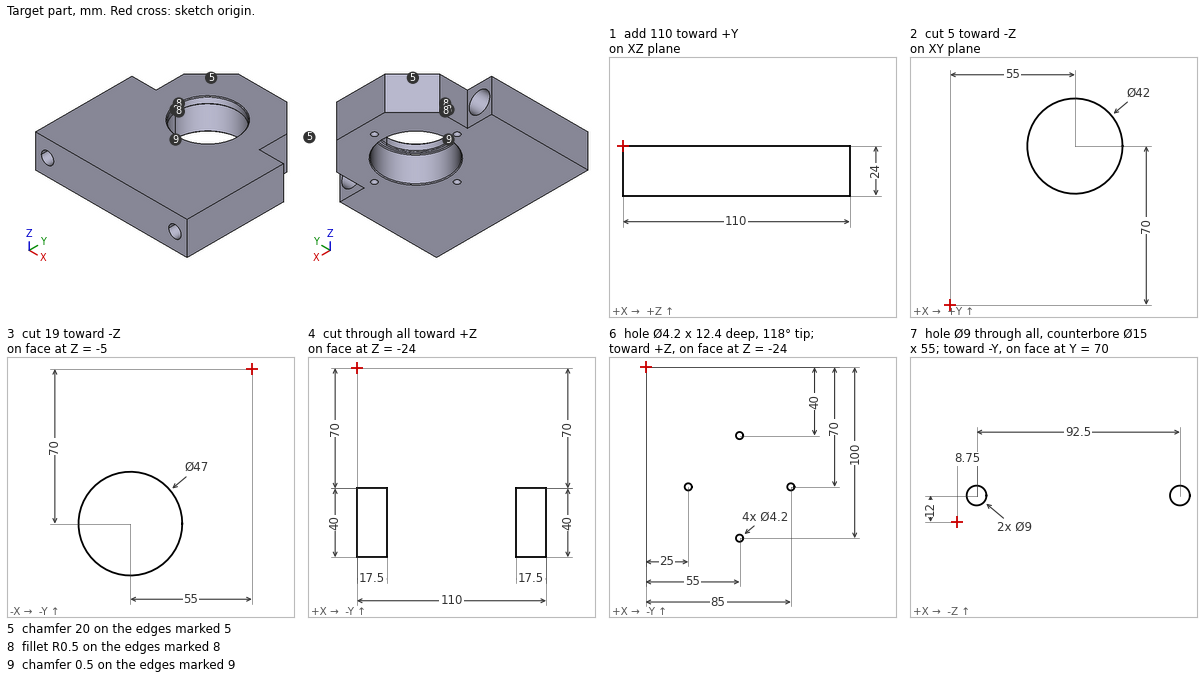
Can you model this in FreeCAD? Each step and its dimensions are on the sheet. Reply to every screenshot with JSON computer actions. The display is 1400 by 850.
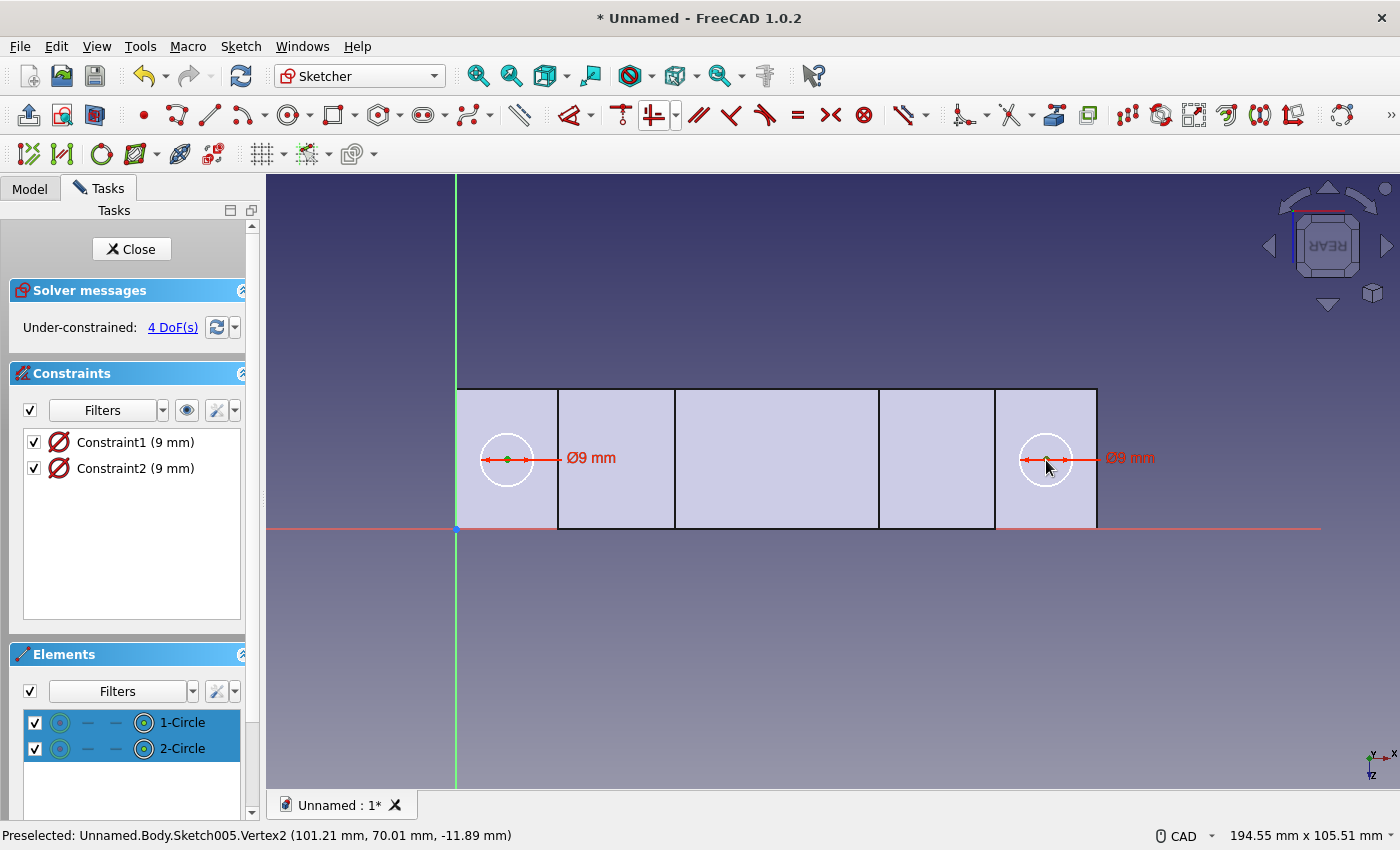
{"action": "left_click", "coordinate": [676, 116]}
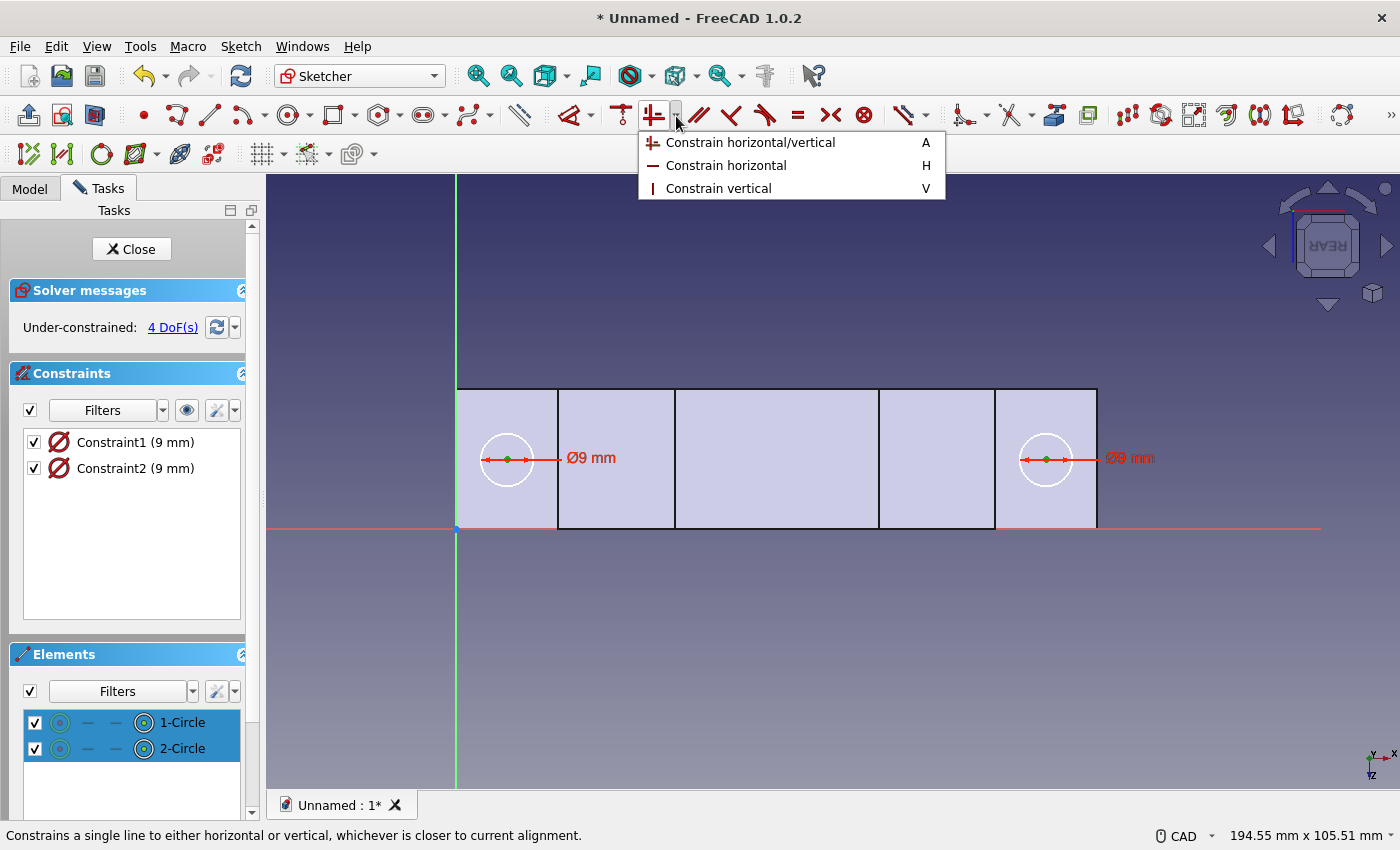
{"action": "left_click", "coordinate": [792, 166]}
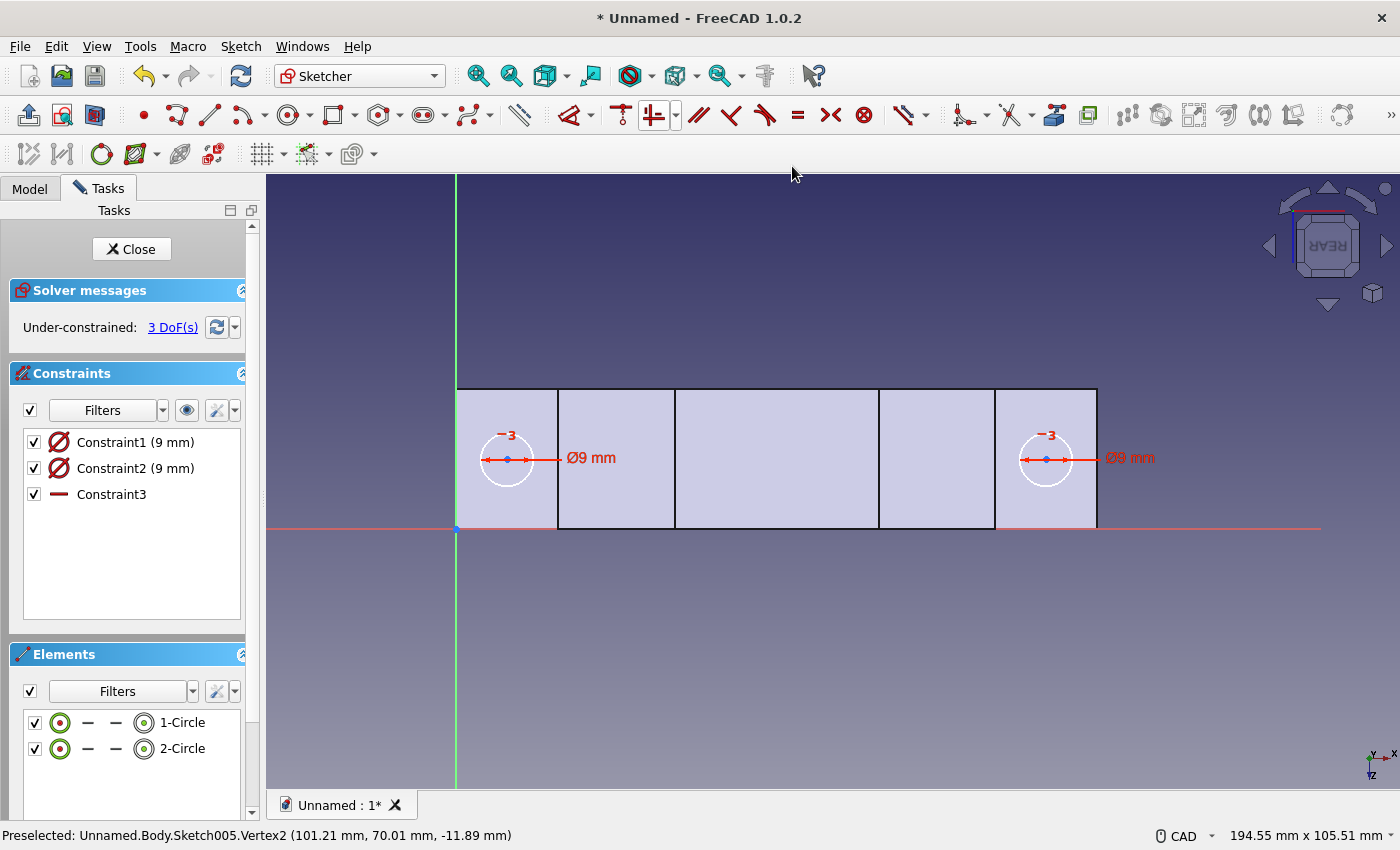
{"action": "left_click", "coordinate": [568, 116]}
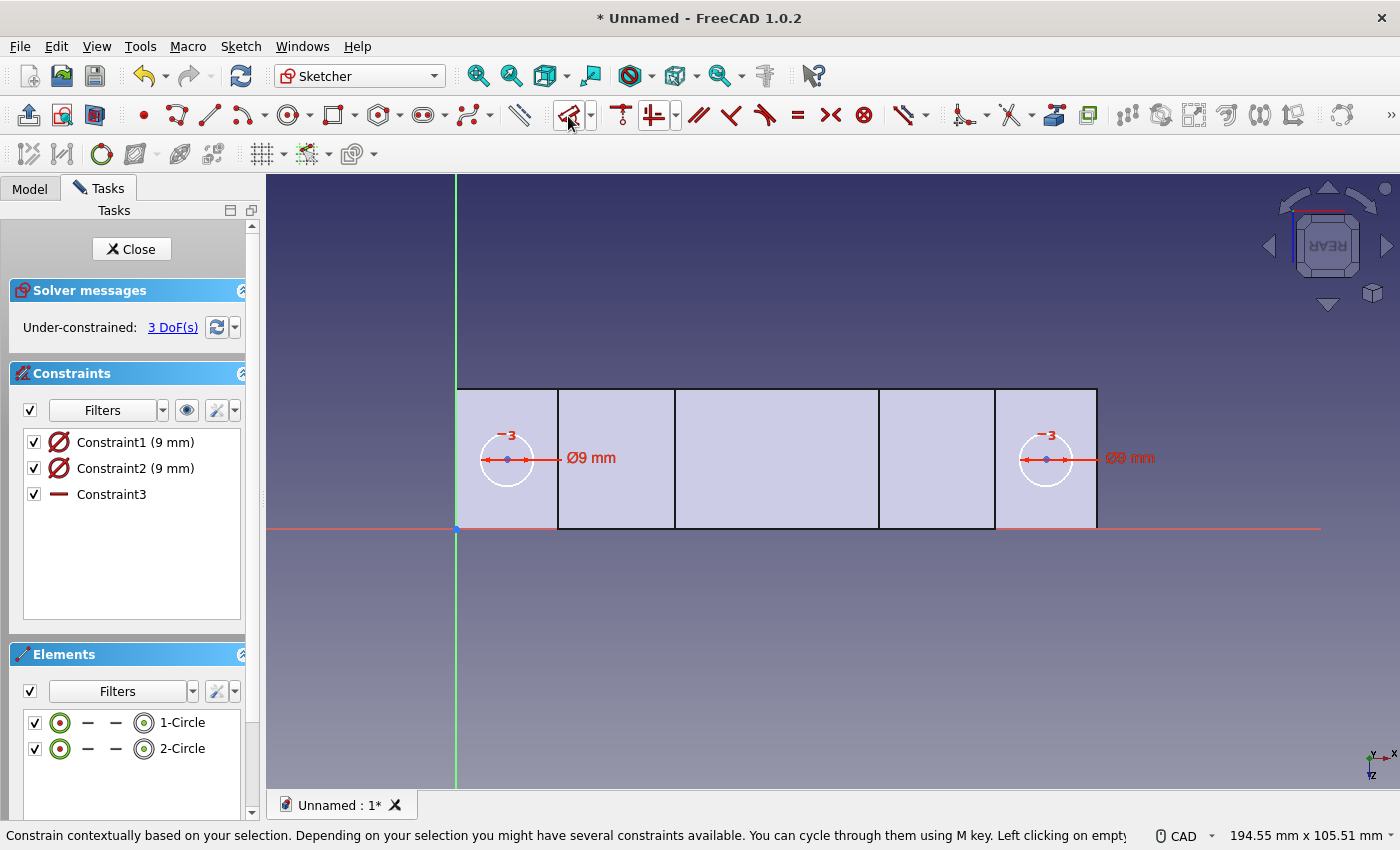
{"action": "left_click", "coordinate": [507, 460]}
{"action": "left_click", "coordinate": [422, 495]}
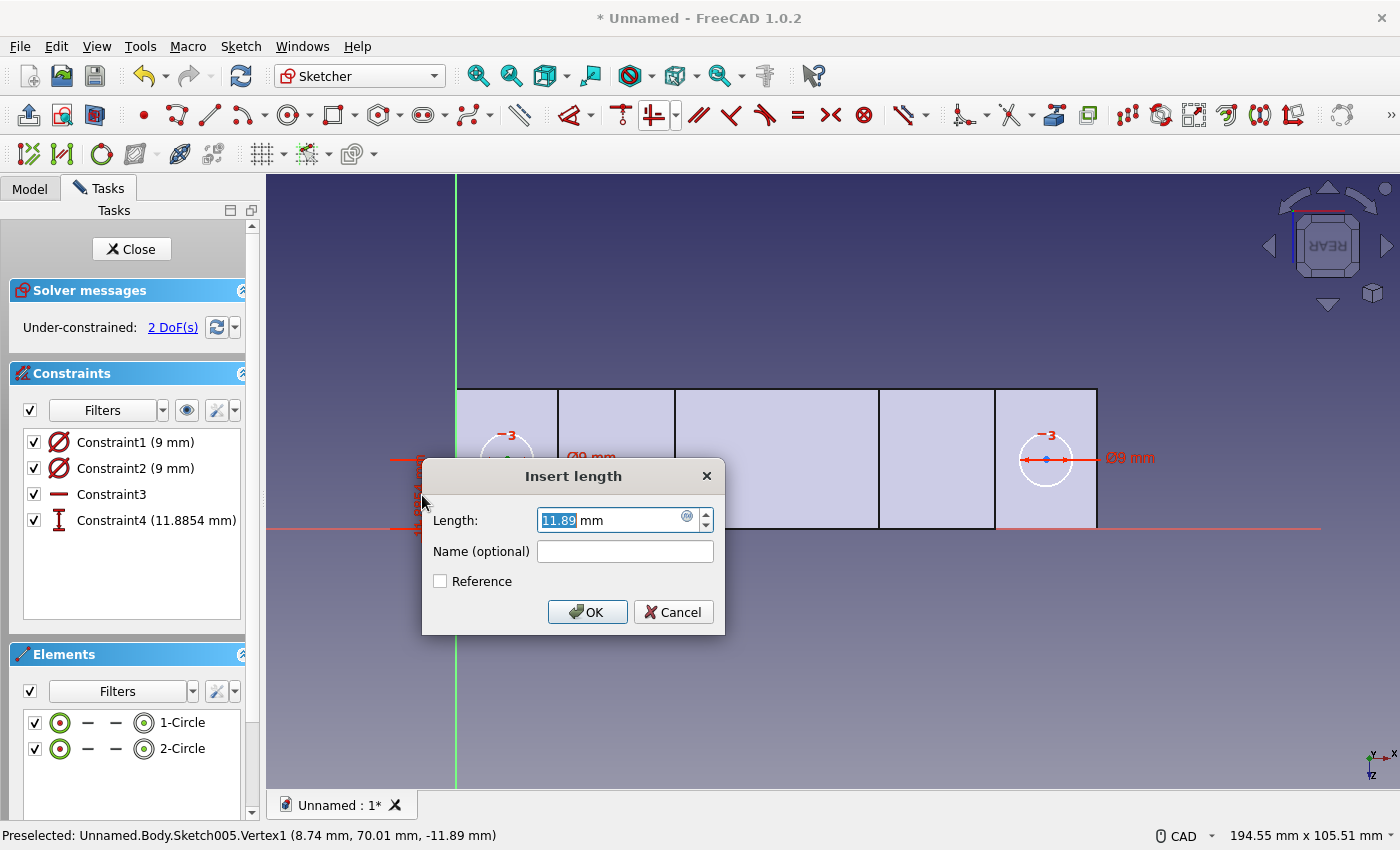
{"action": "type", "text": "12"}
{"action": "key", "text": "Return"}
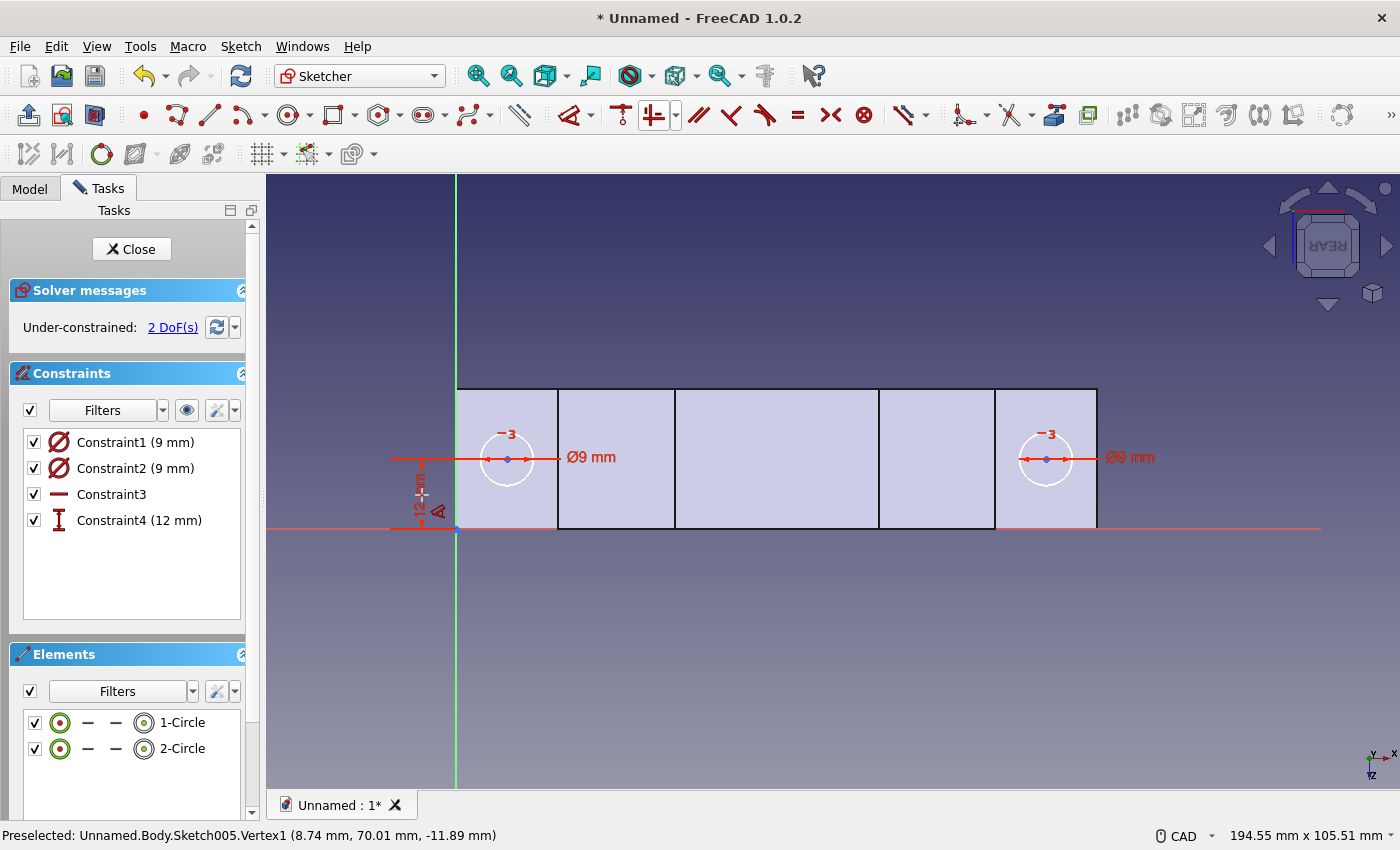
{"action": "left_click", "coordinate": [507, 459]}
{"action": "left_click", "coordinate": [482, 563]}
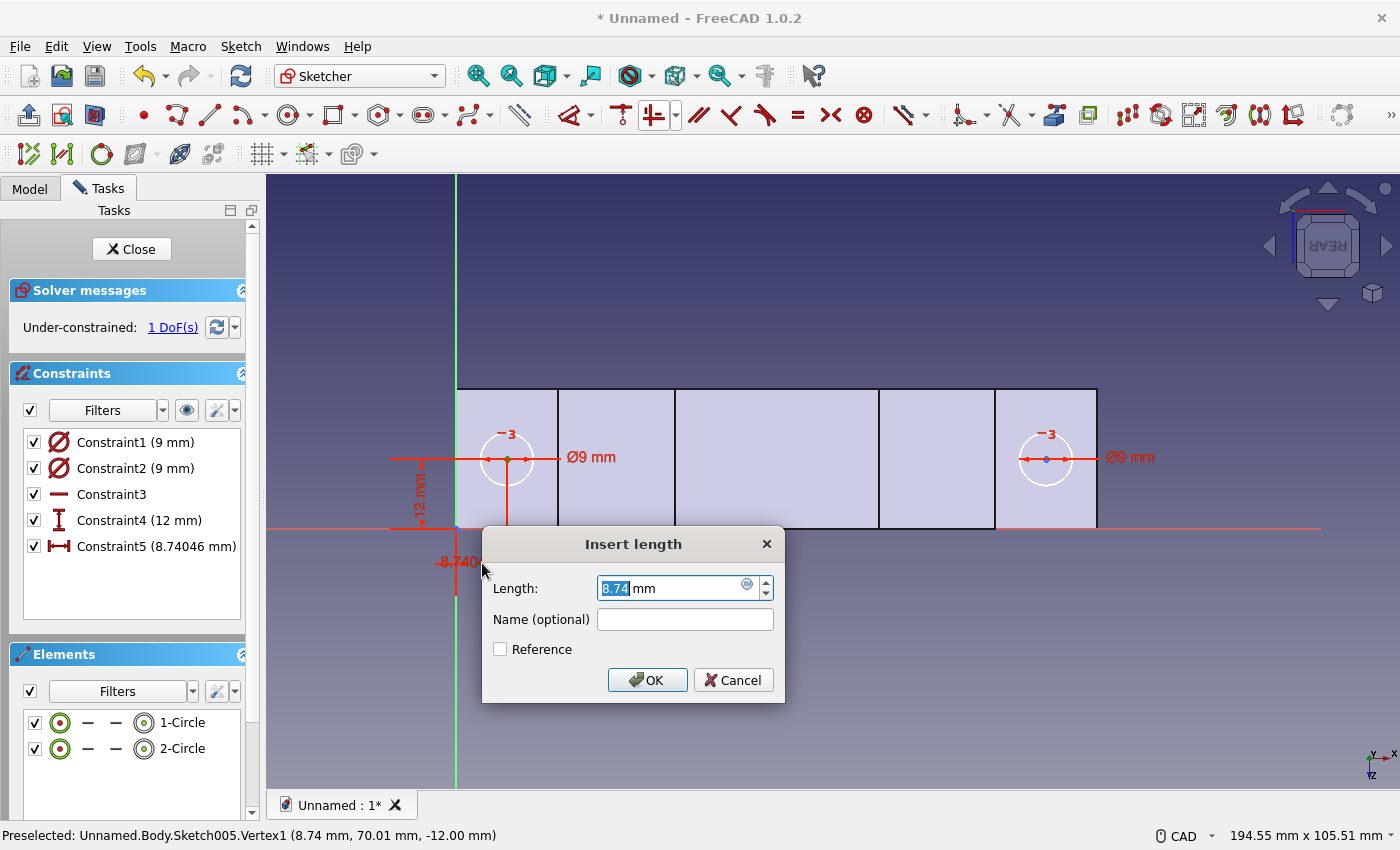
{"action": "type", "text": "8.75"}
{"action": "key", "text": "Return"}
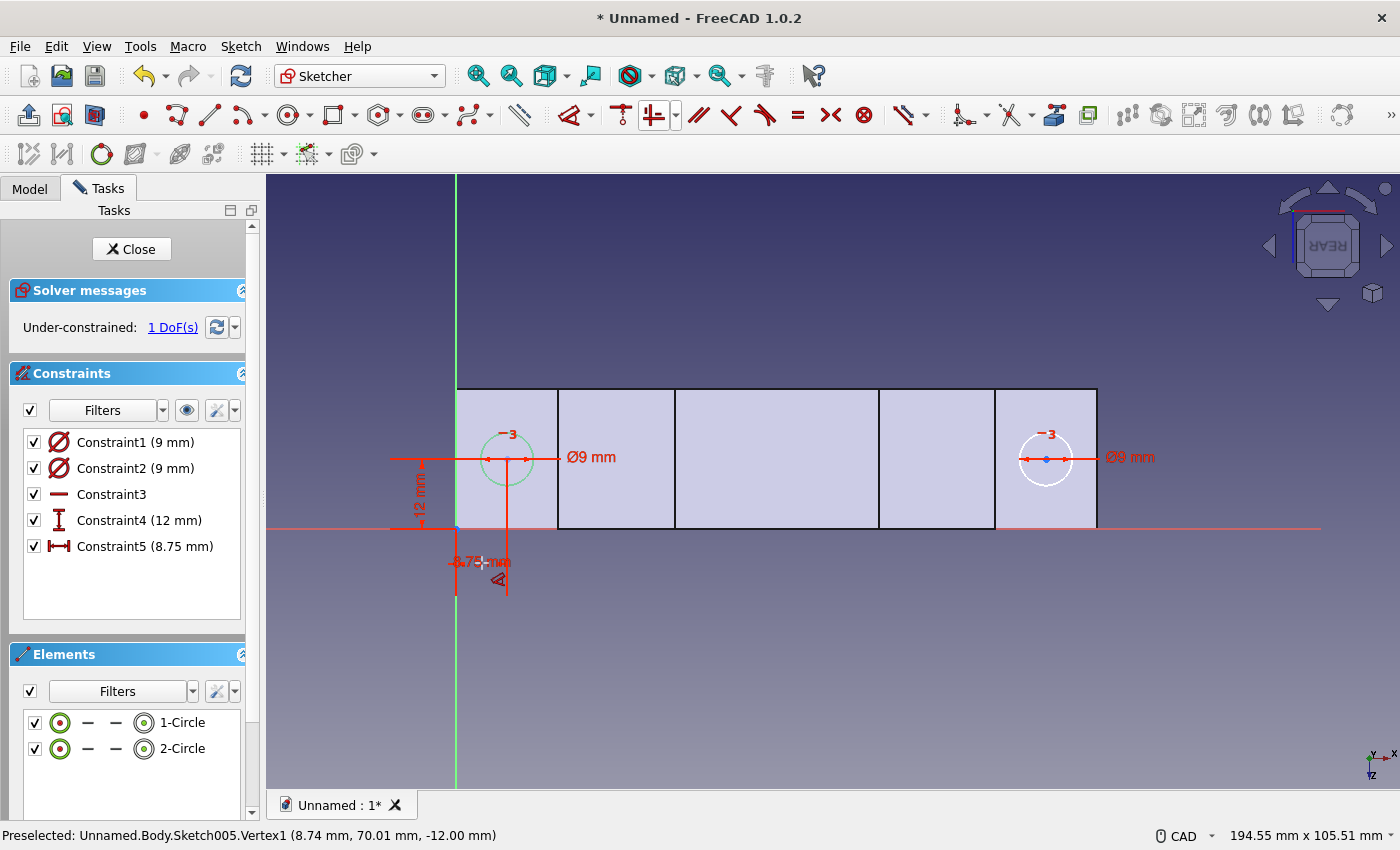
{"action": "left_click", "coordinate": [507, 459]}